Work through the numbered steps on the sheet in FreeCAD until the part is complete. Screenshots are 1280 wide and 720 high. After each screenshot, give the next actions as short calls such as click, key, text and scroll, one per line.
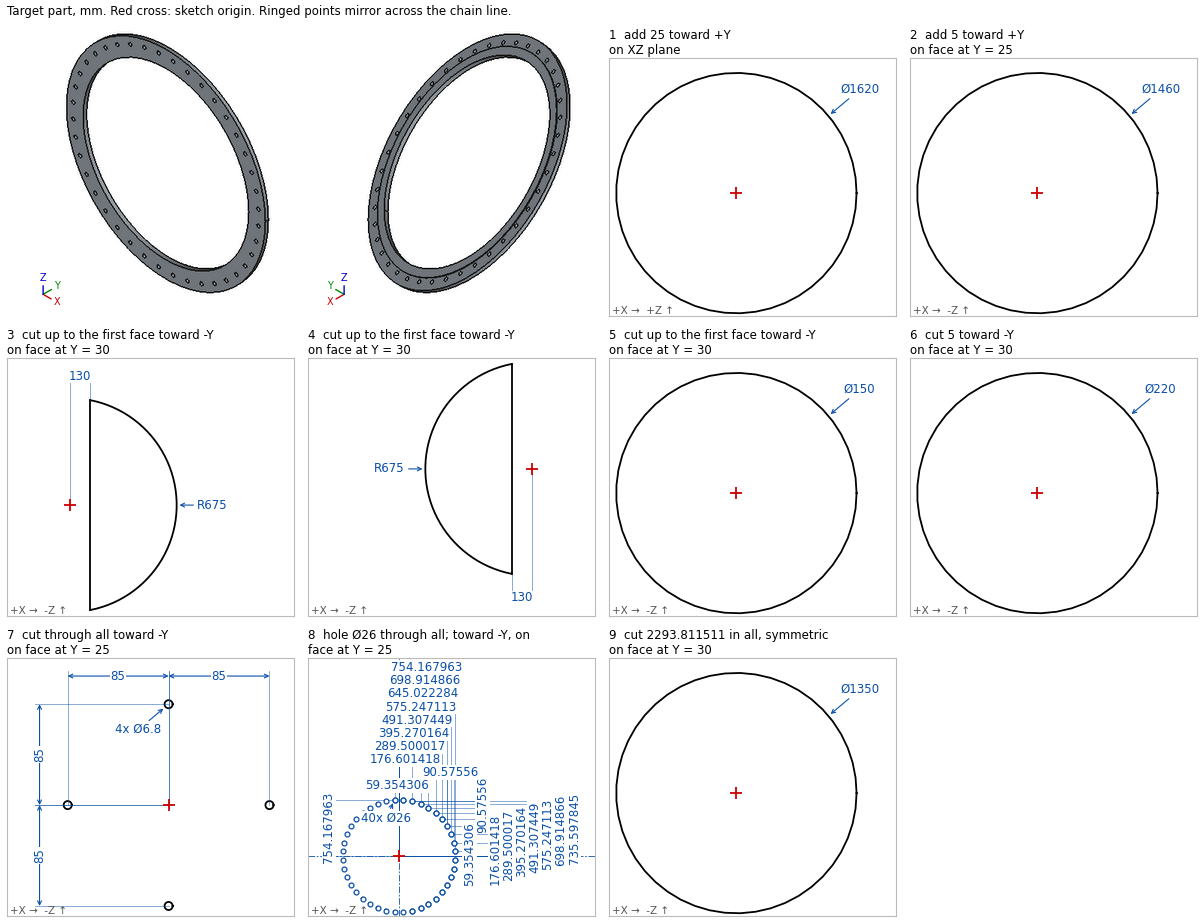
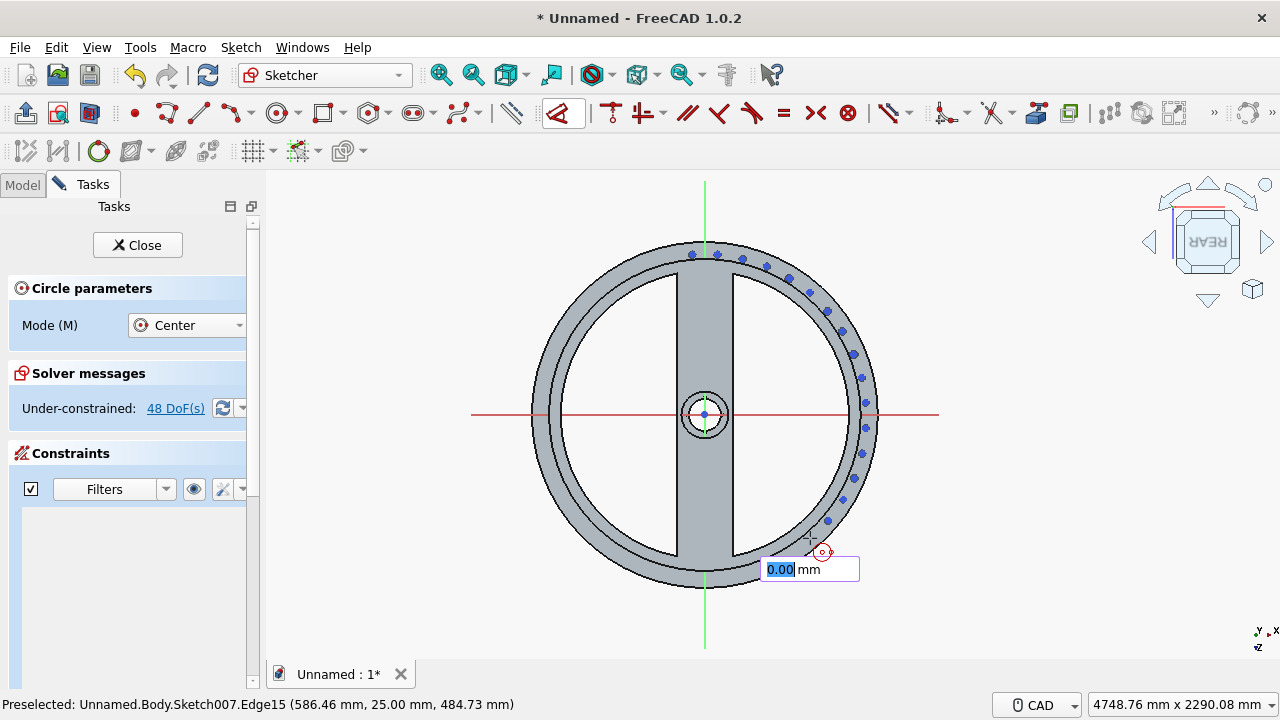
scroll(812, 536, up, 9)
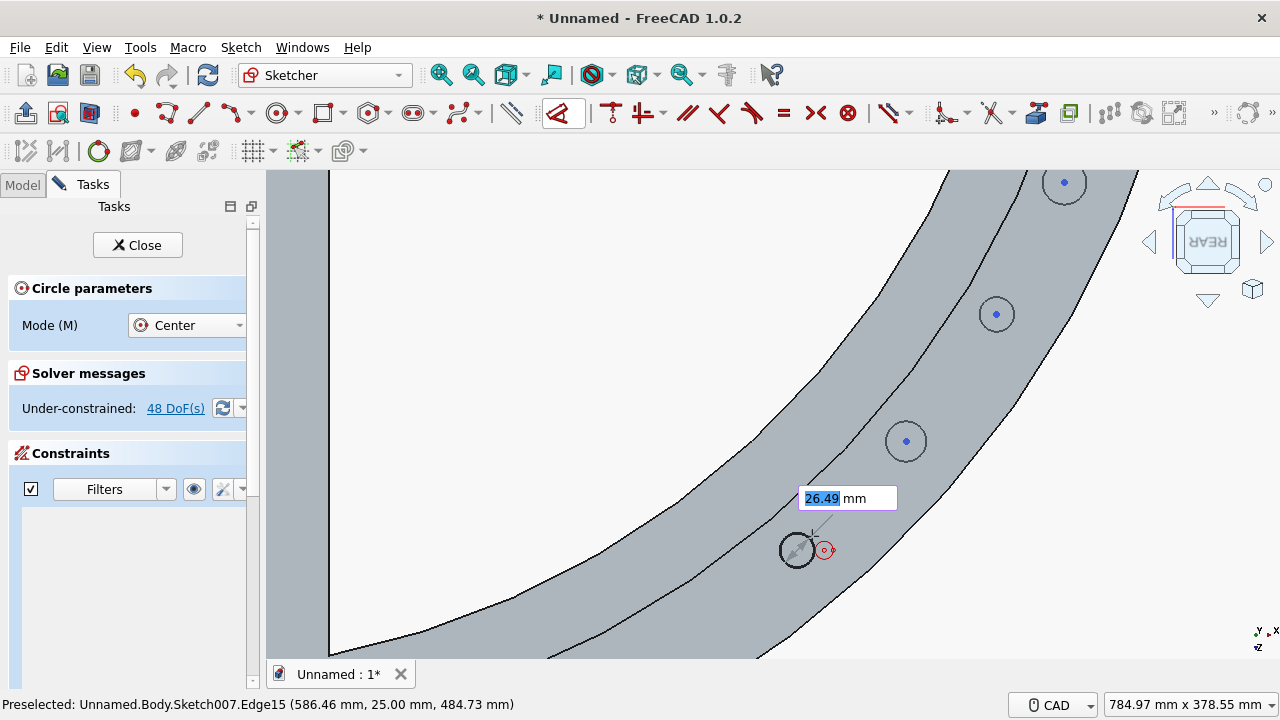
click(808, 531)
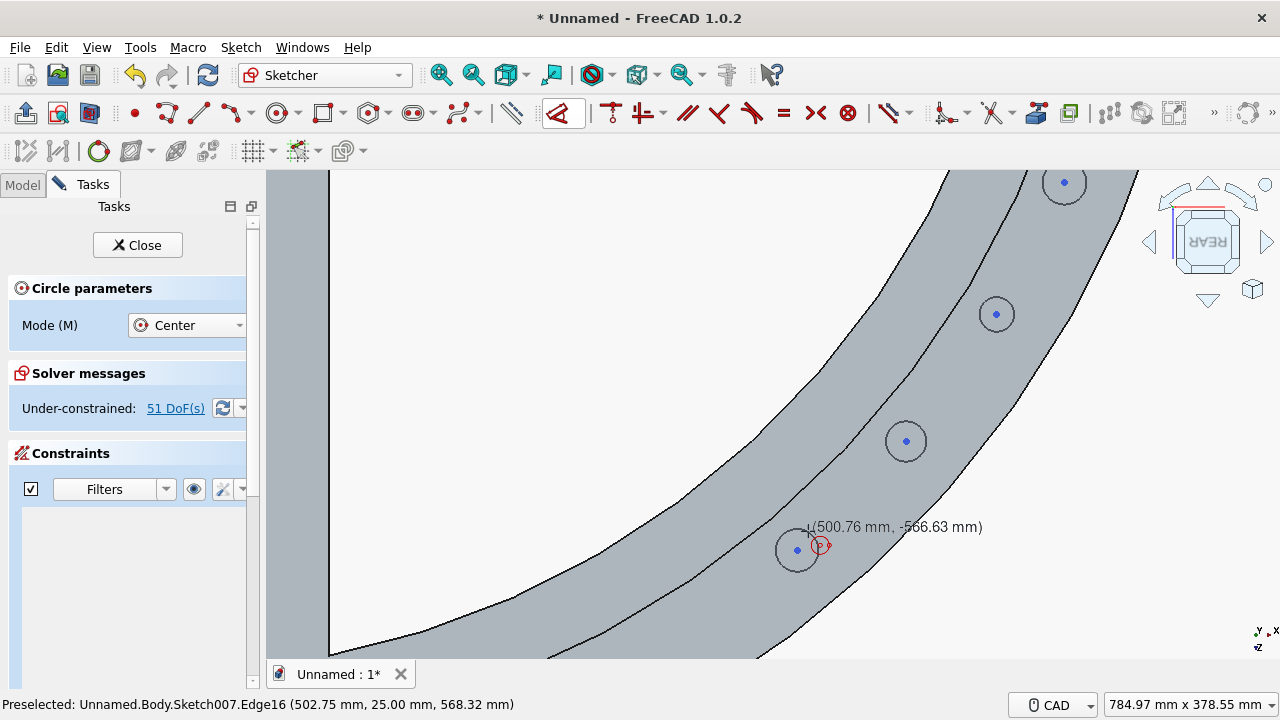
scroll(812, 536, down, 9)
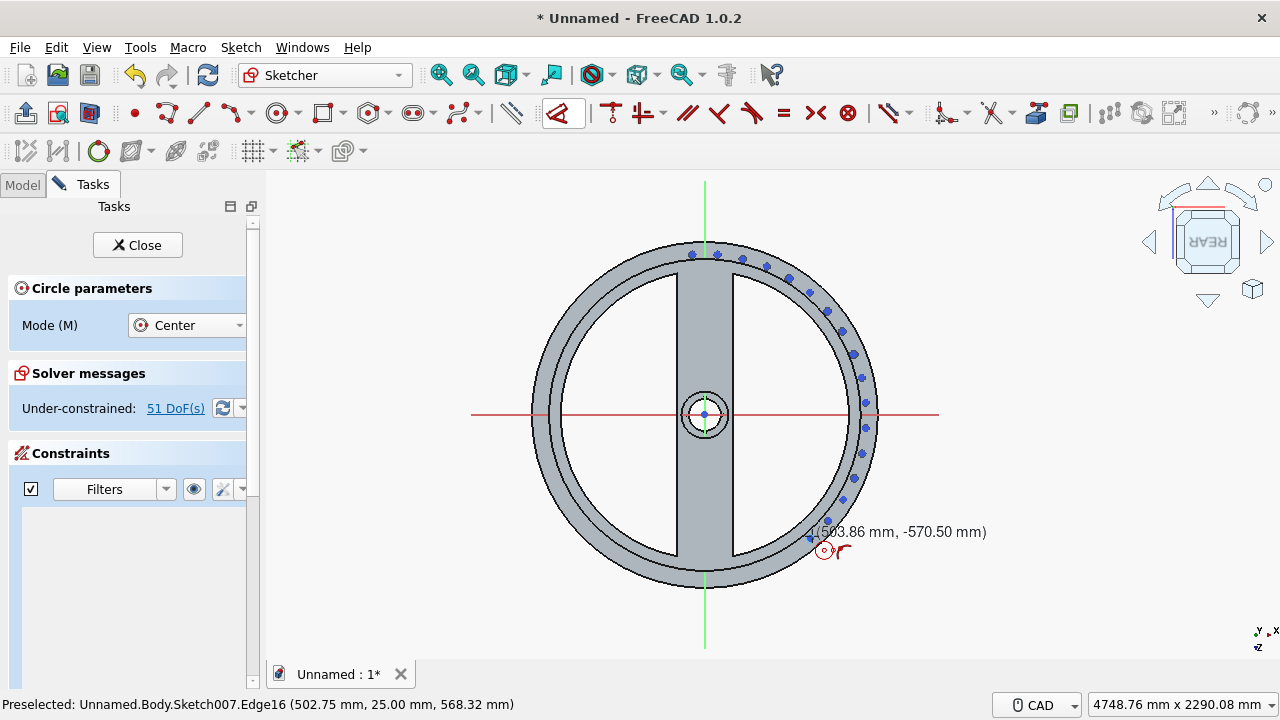
scroll(789, 553, up, 11)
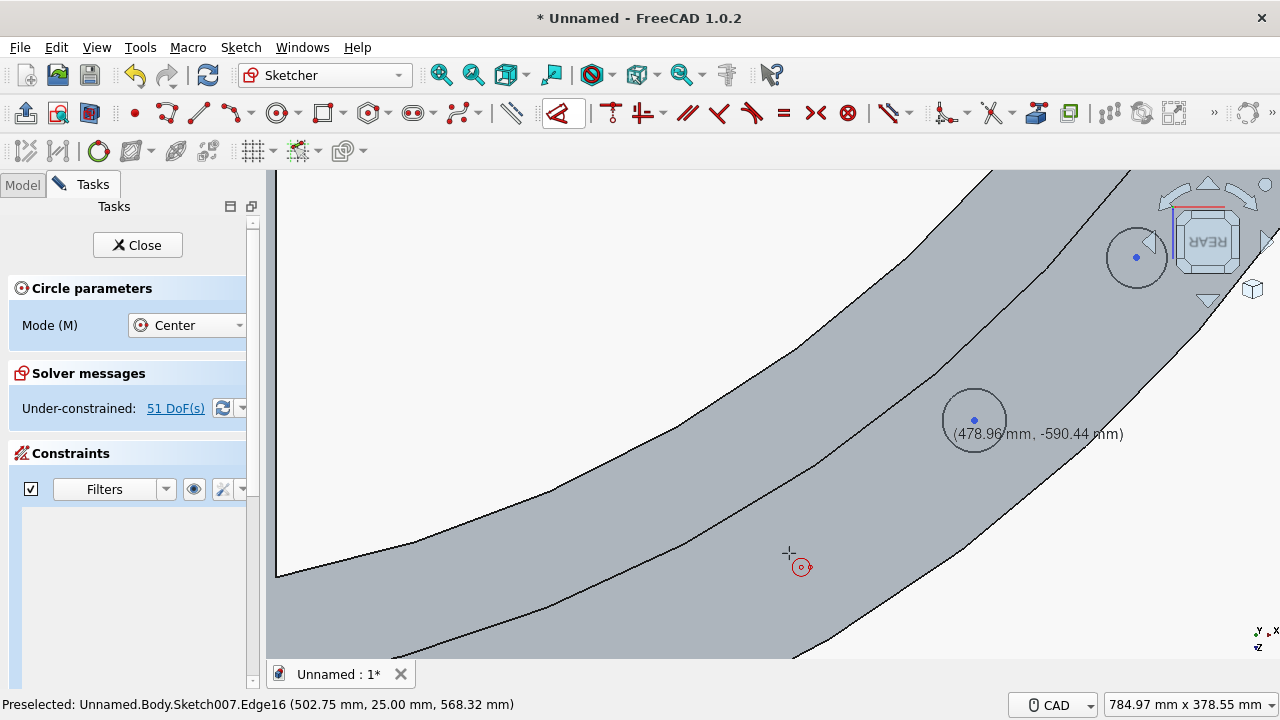
scroll(789, 553, down, 11)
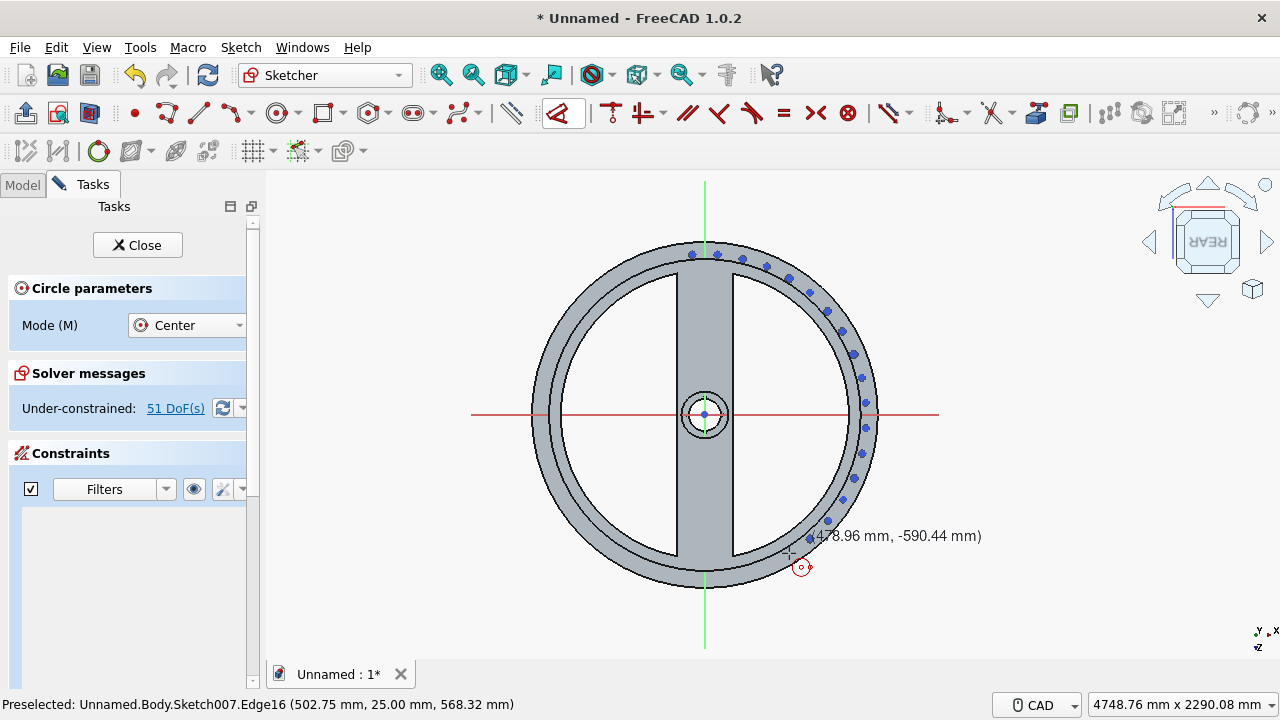
click(789, 553)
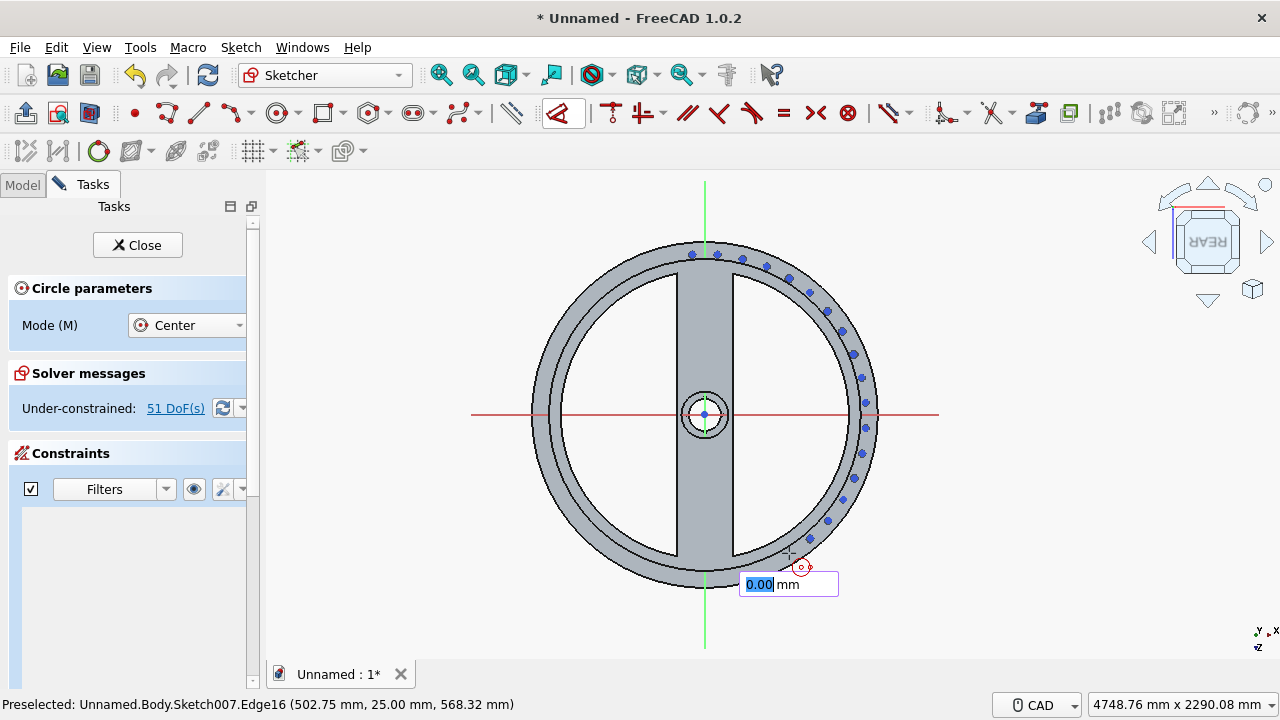
scroll(791, 551, up, 9)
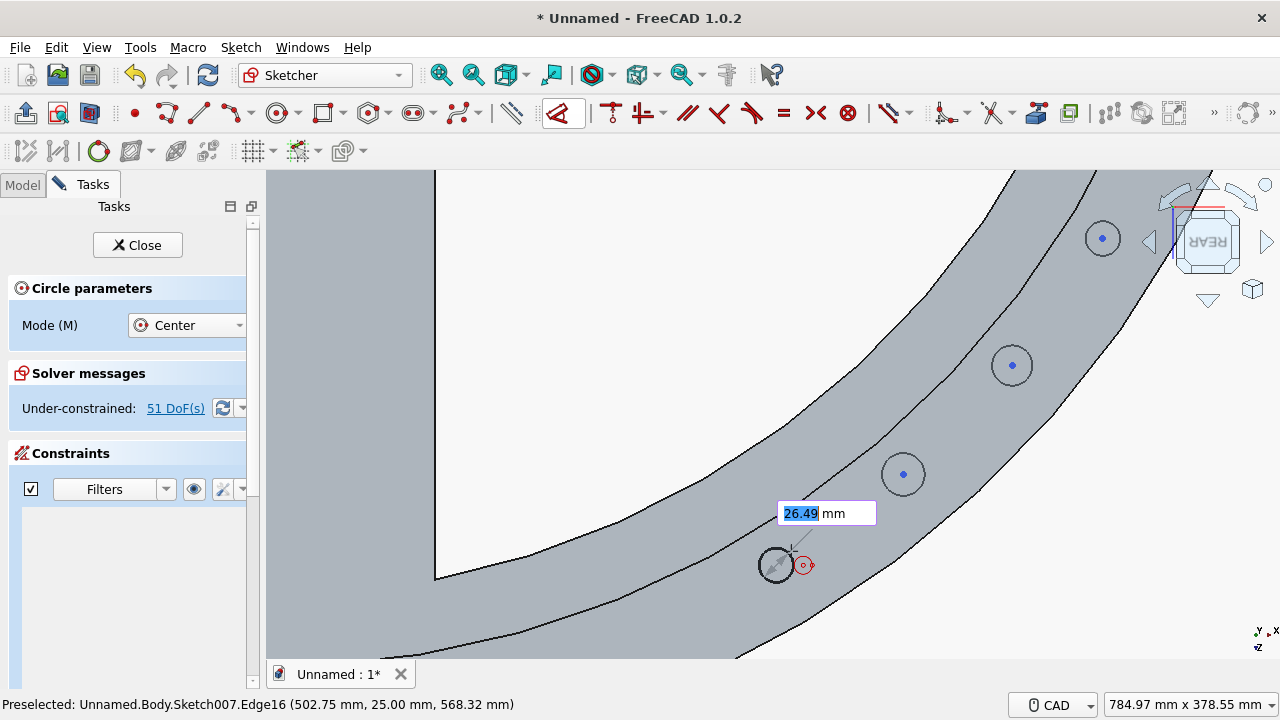
click(790, 545)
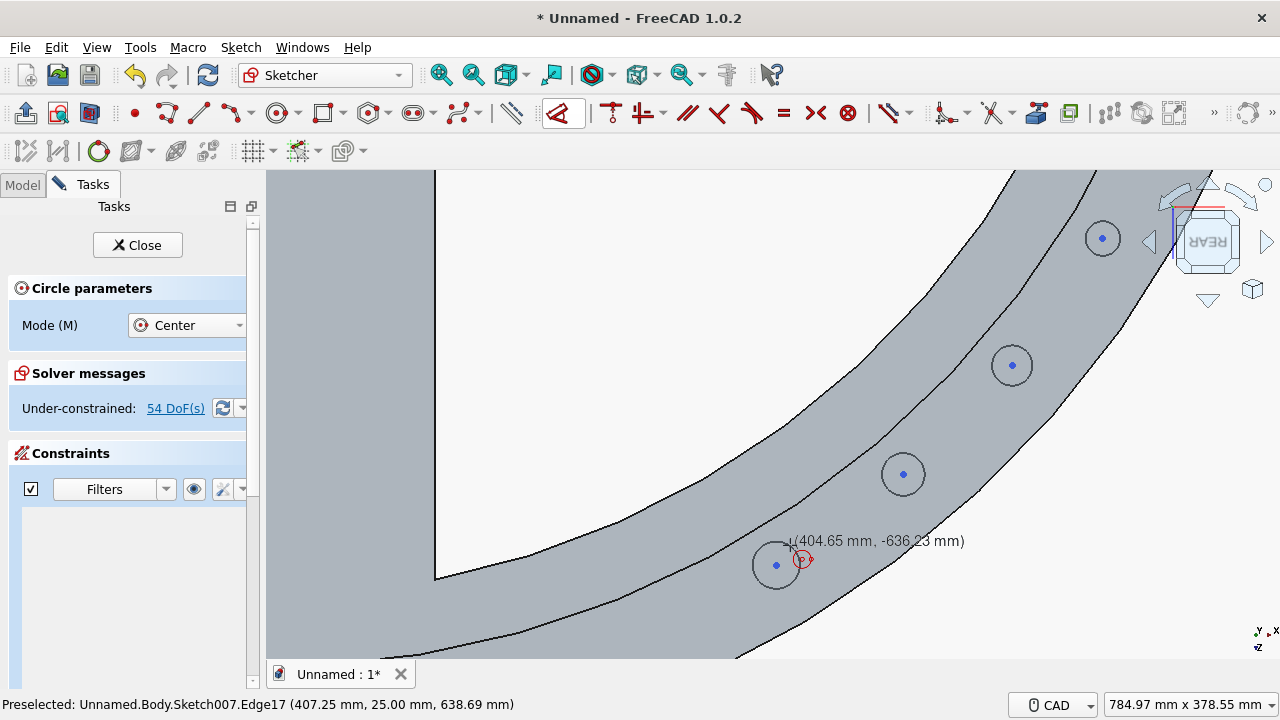
scroll(641, 627, up, 2)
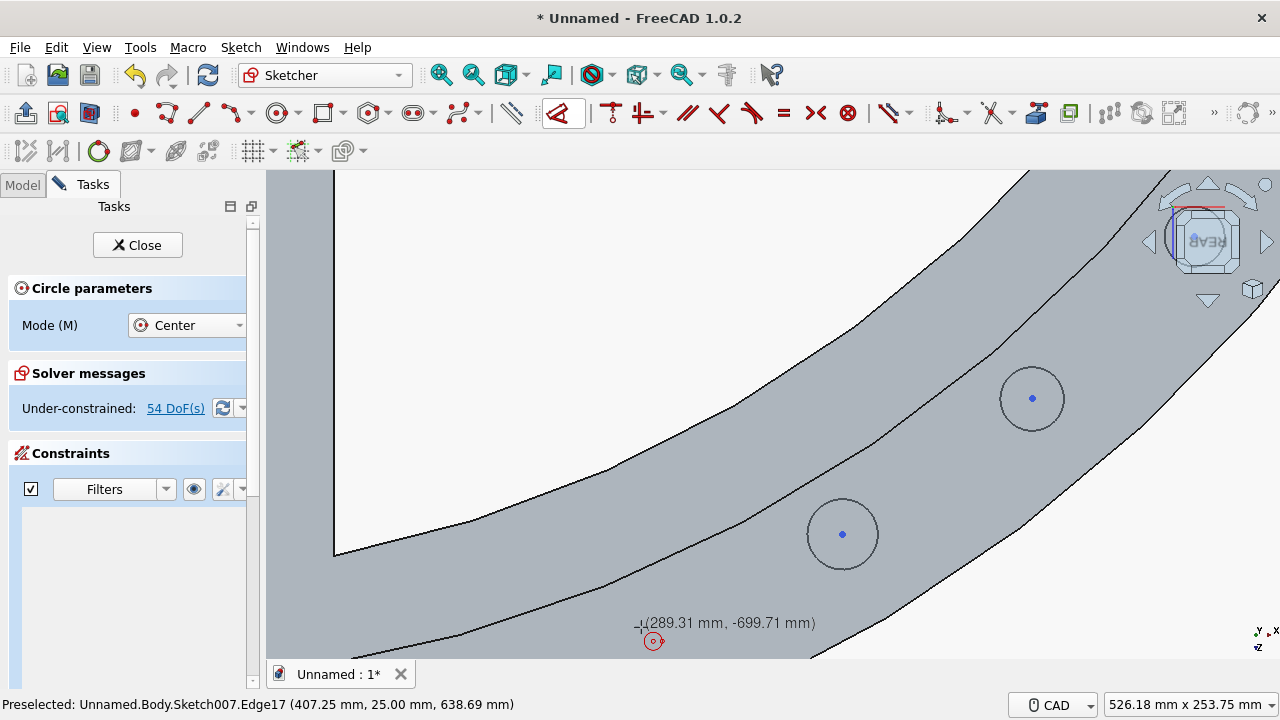
scroll(782, 556, down, 11)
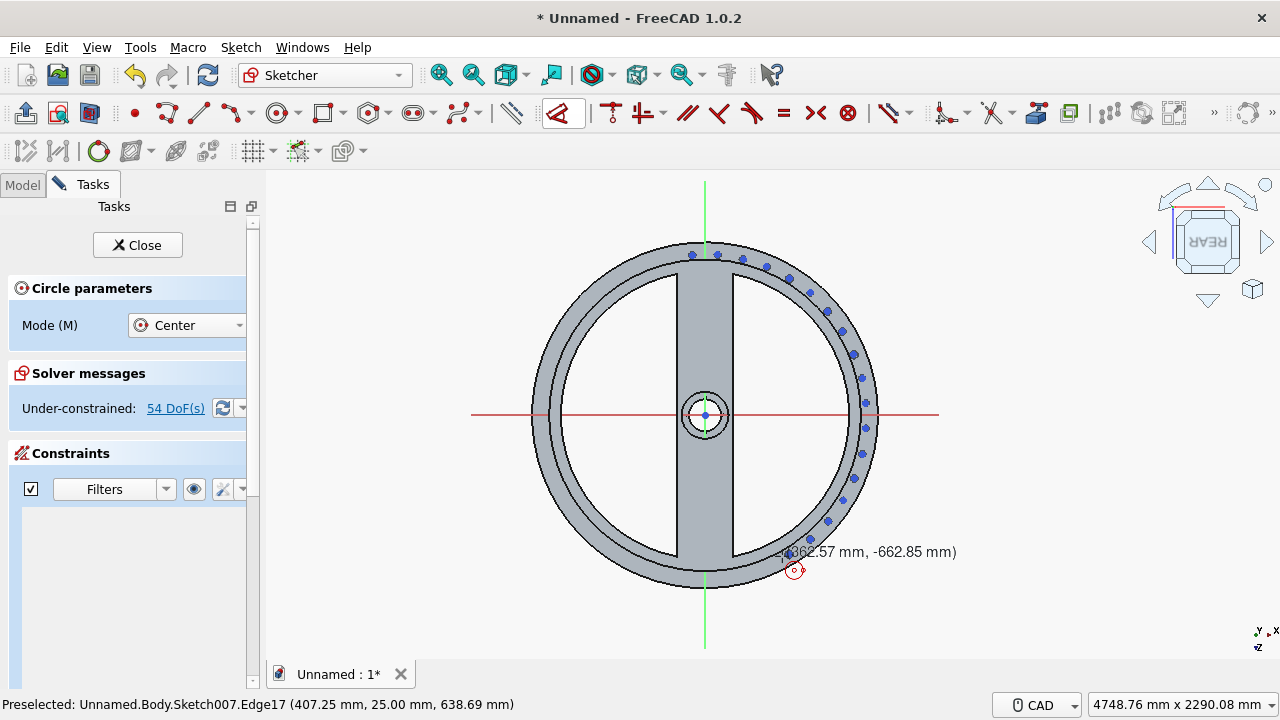
click(767, 565)